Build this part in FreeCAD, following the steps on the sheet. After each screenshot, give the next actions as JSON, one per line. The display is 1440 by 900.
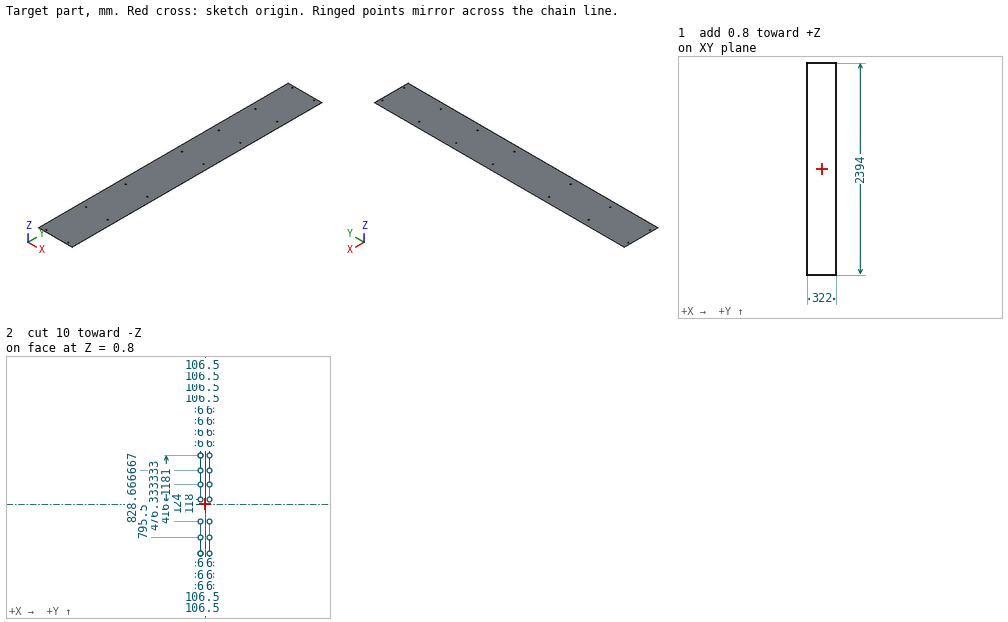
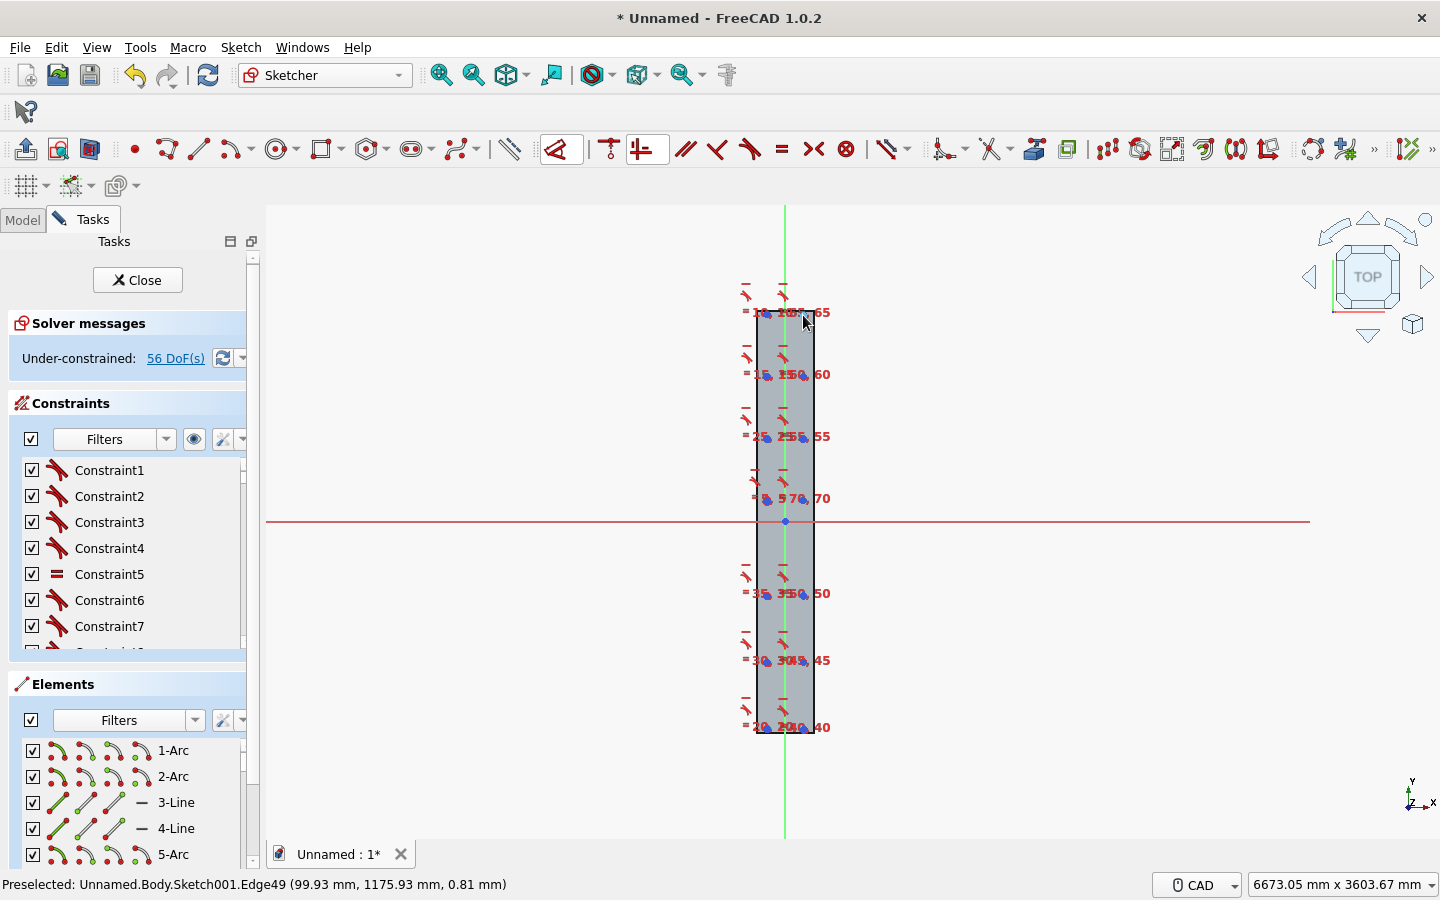
{"action": "scroll", "coordinate": [802, 500], "scroll_direction": "up", "scroll_amount": 14}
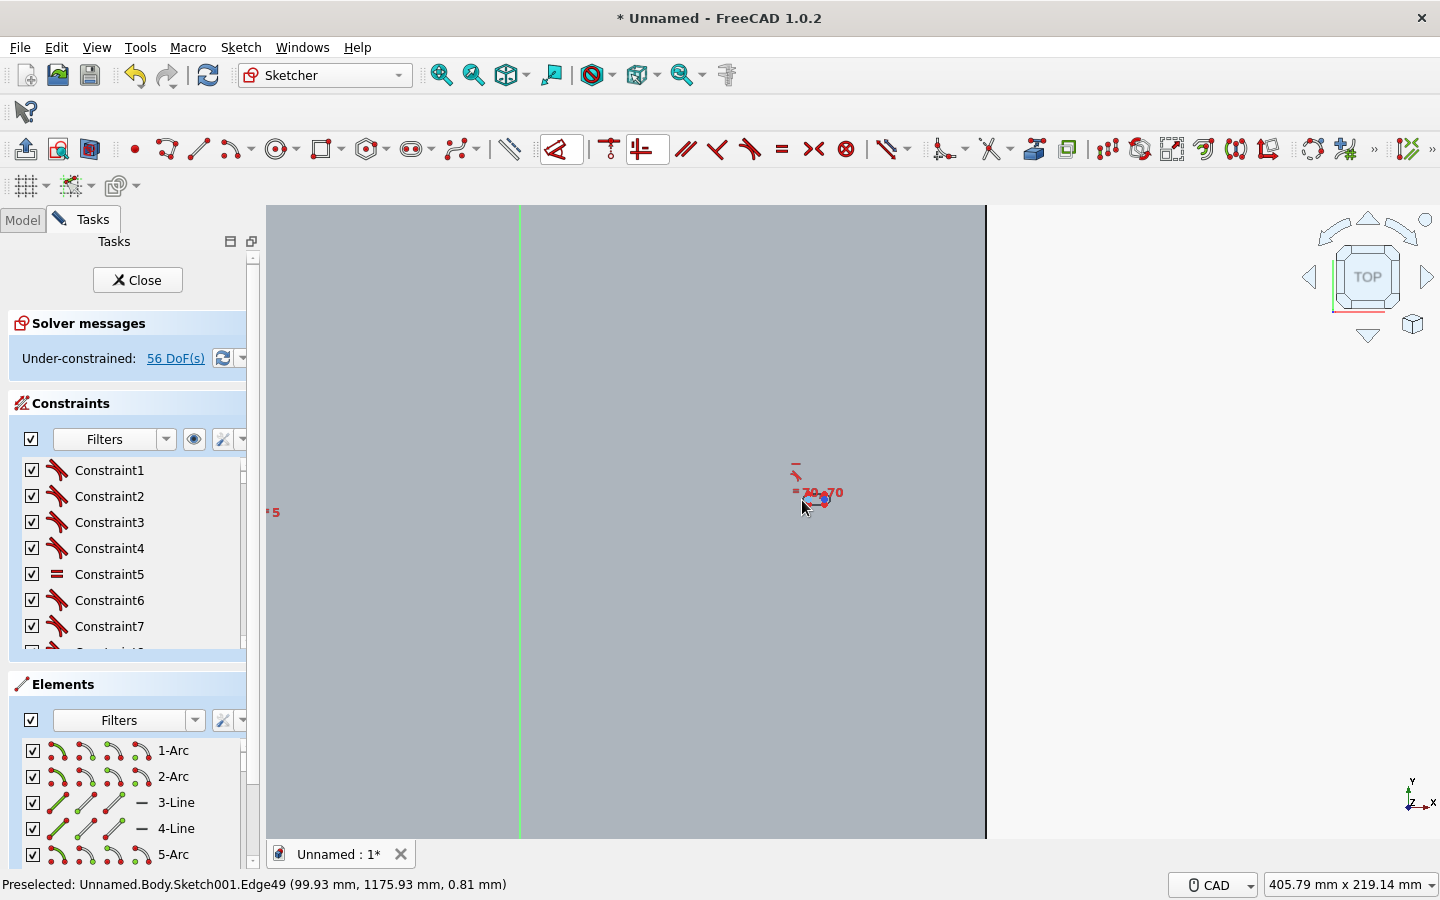
{"action": "left_click", "coordinate": [803, 500]}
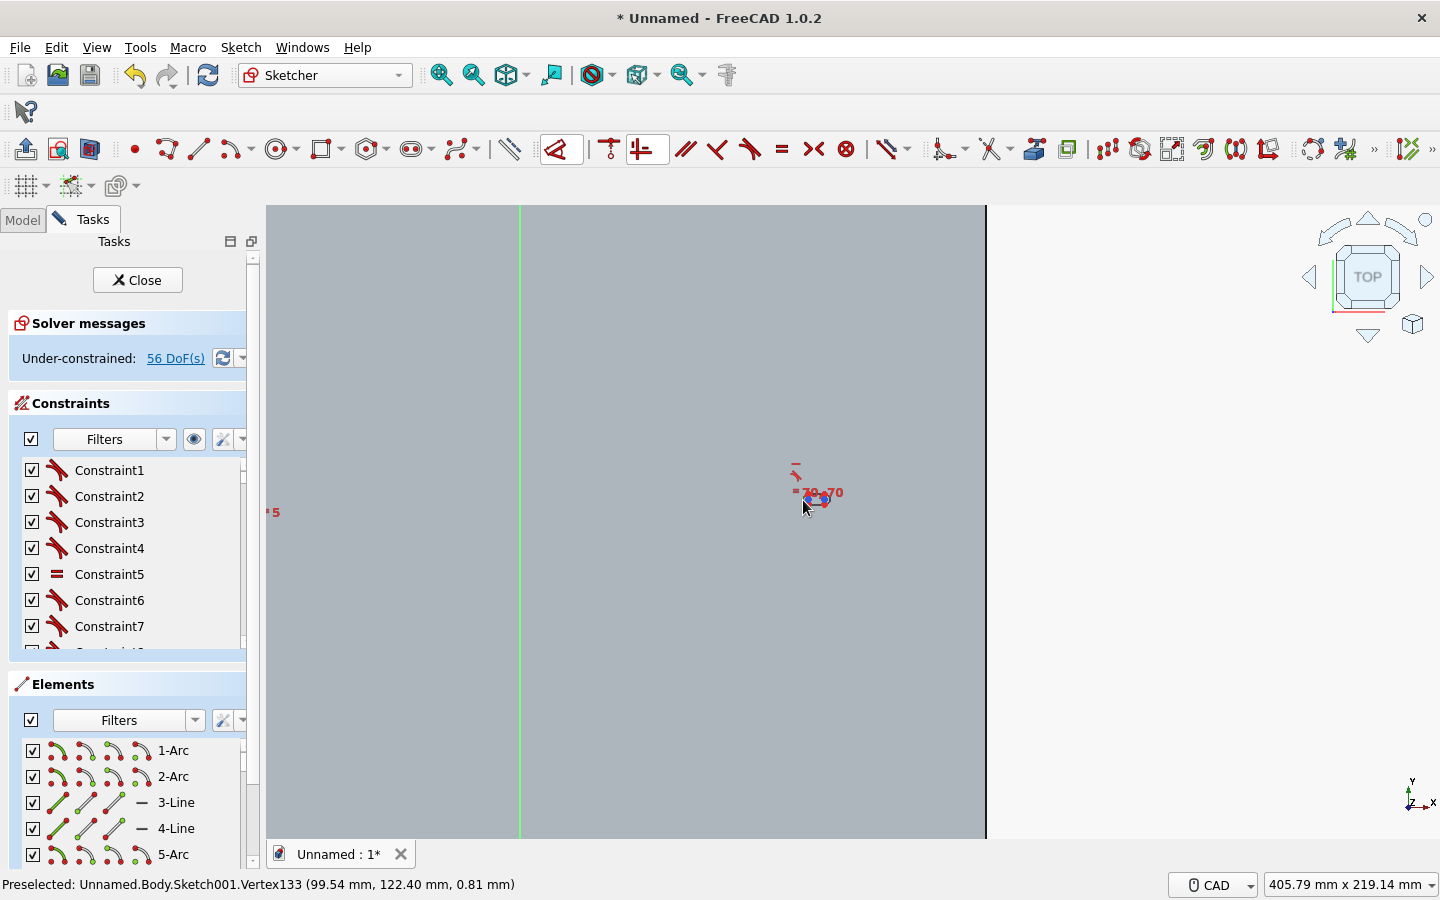
{"action": "left_click", "coordinate": [782, 150]}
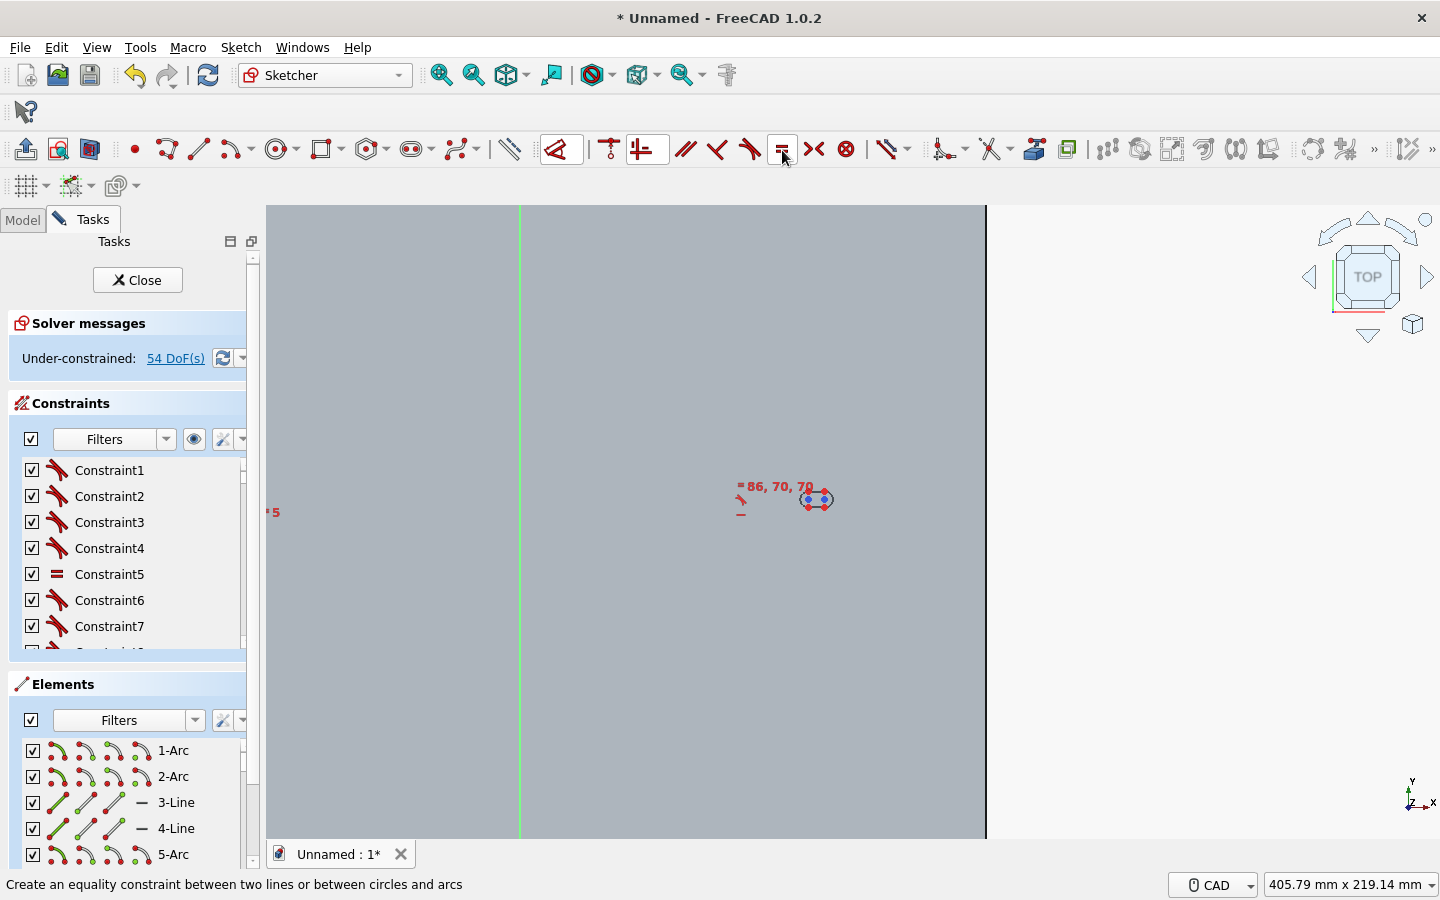
{"action": "scroll", "coordinate": [802, 501], "scroll_direction": "down", "scroll_amount": 14}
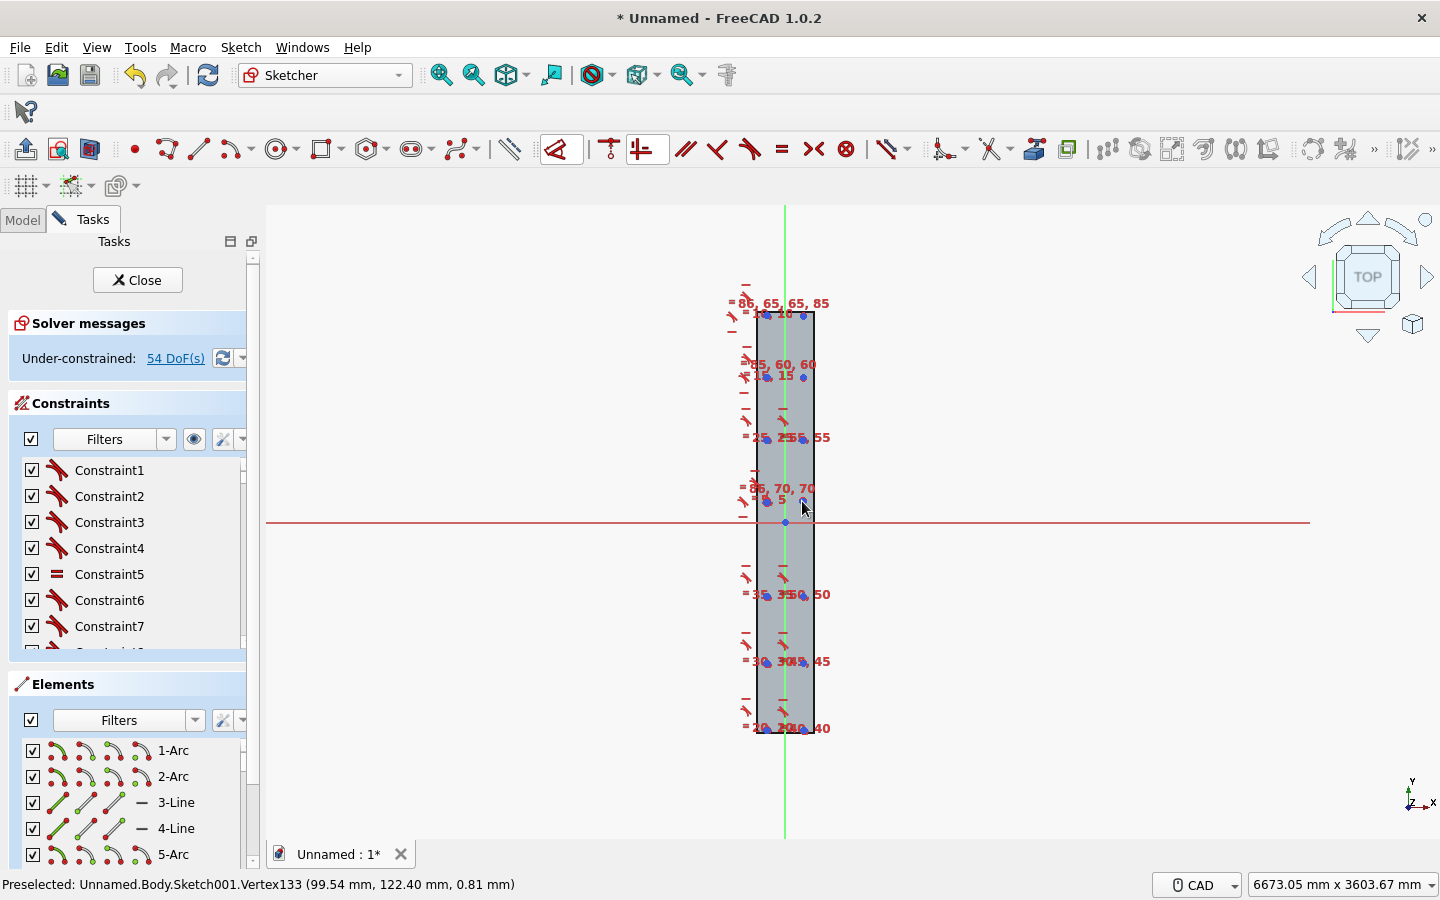
{"action": "scroll", "coordinate": [766, 501], "scroll_direction": "up", "scroll_amount": 13}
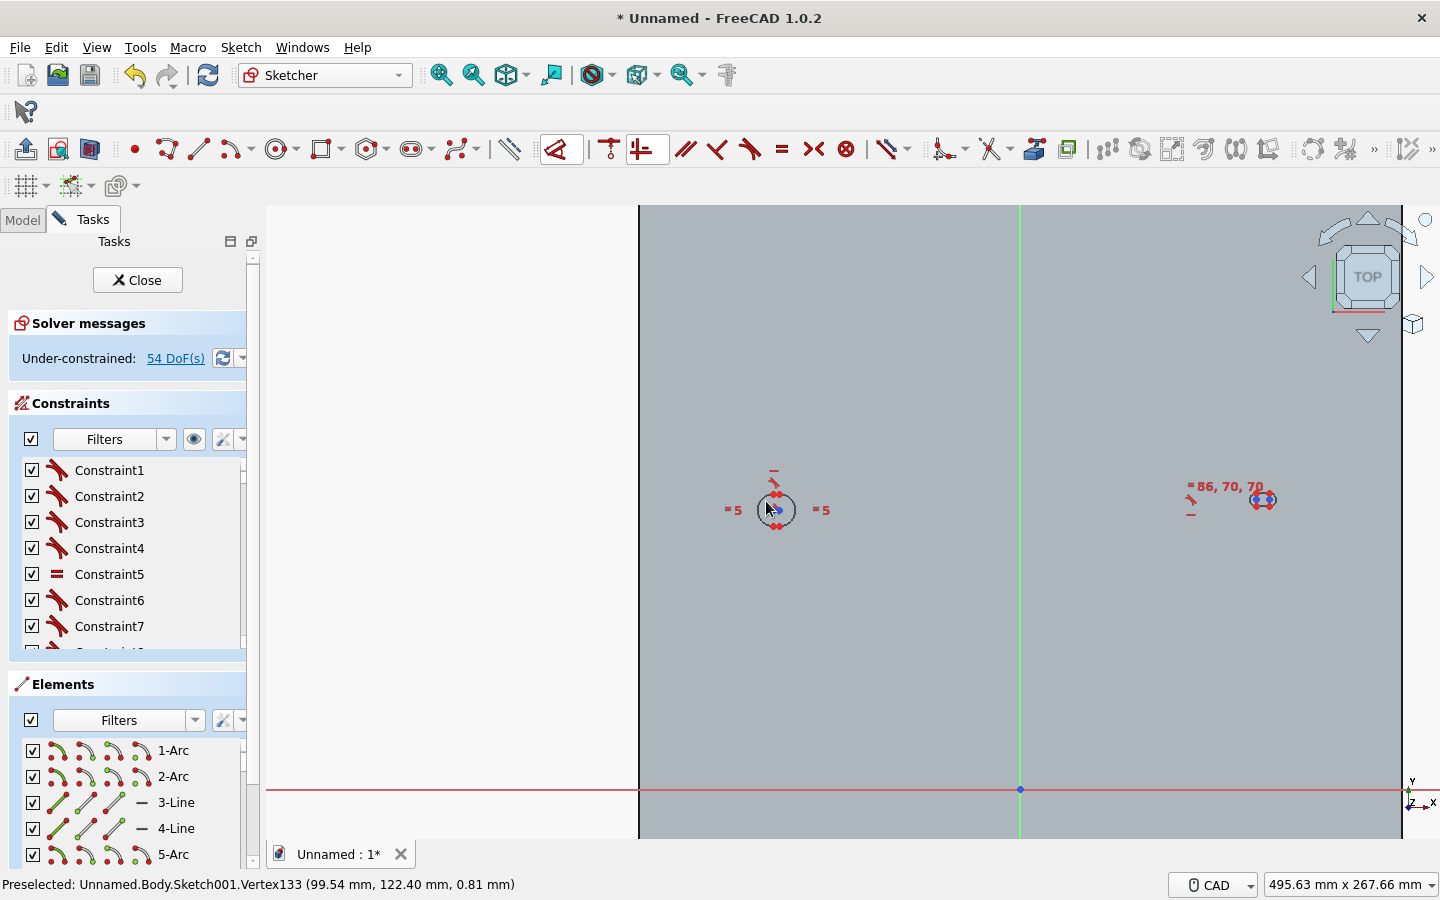
{"action": "left_click", "coordinate": [761, 501]}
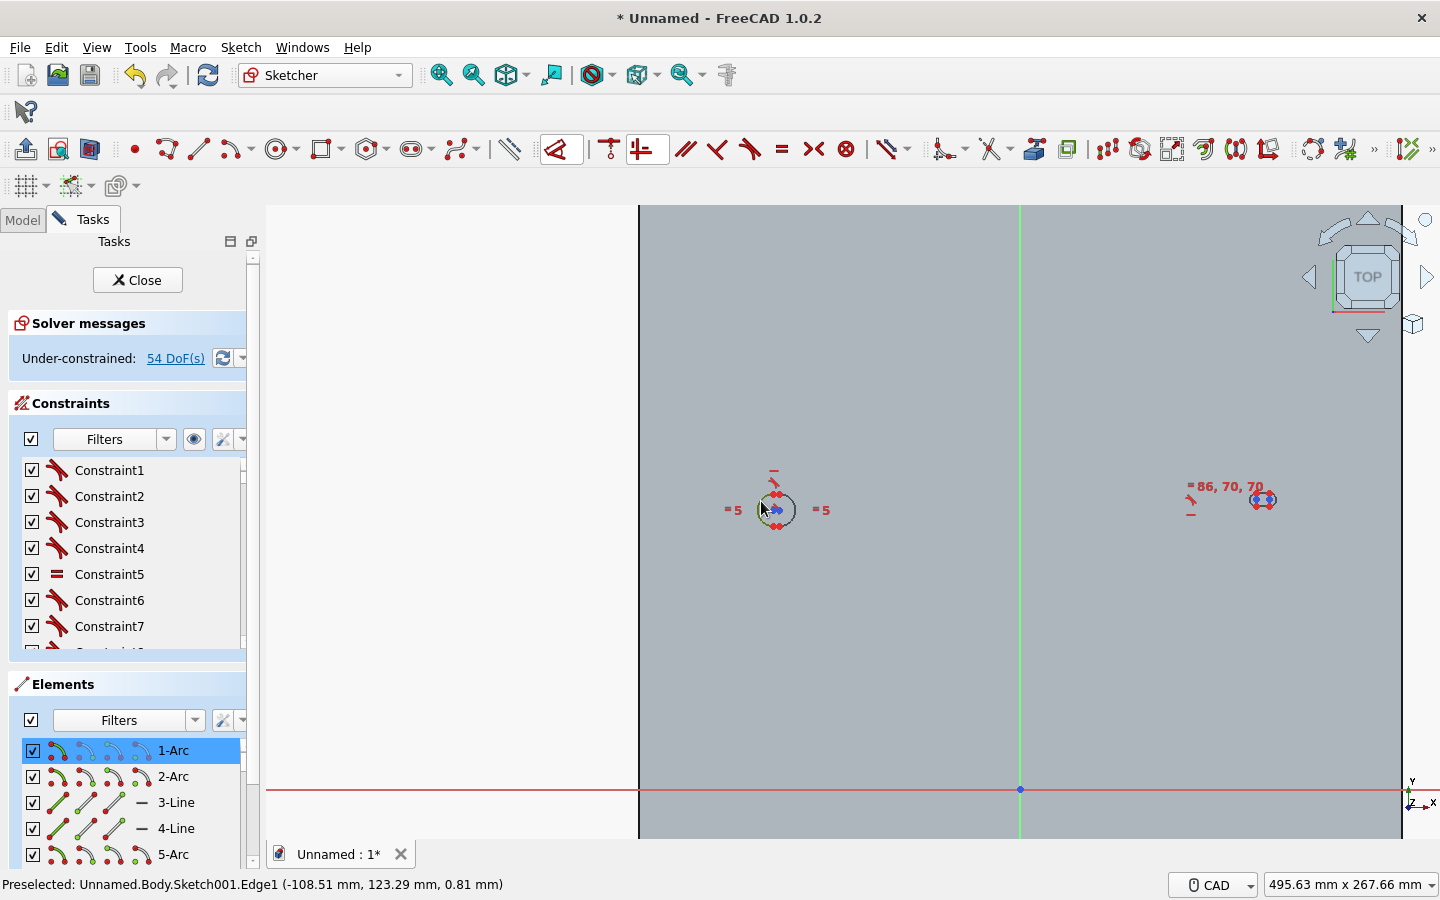
{"action": "scroll", "coordinate": [766, 501], "scroll_direction": "down", "scroll_amount": 13}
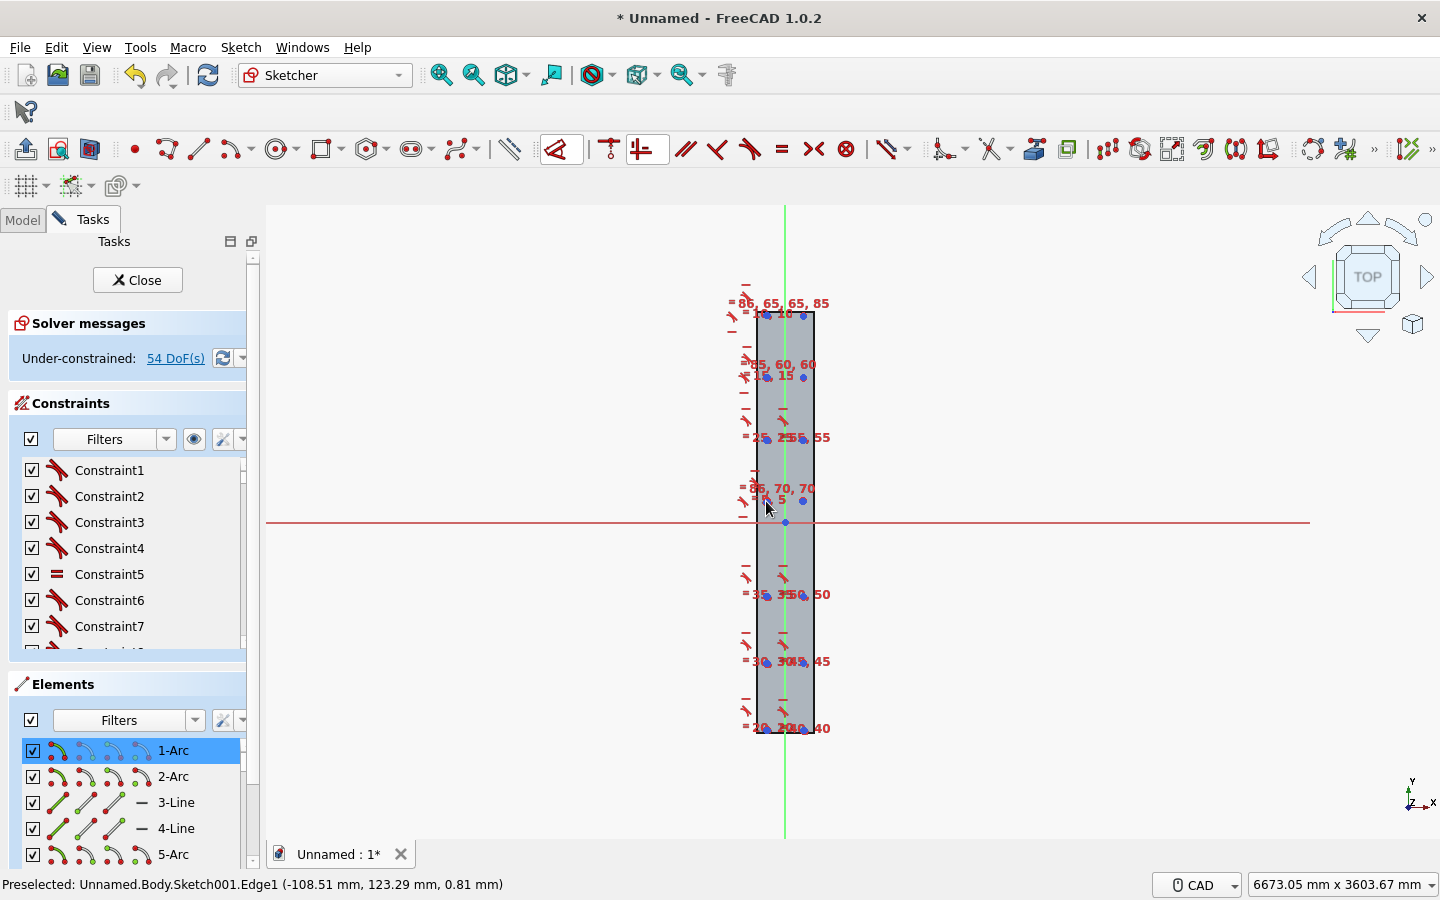
{"action": "scroll", "coordinate": [768, 315], "scroll_direction": "up", "scroll_amount": 14}